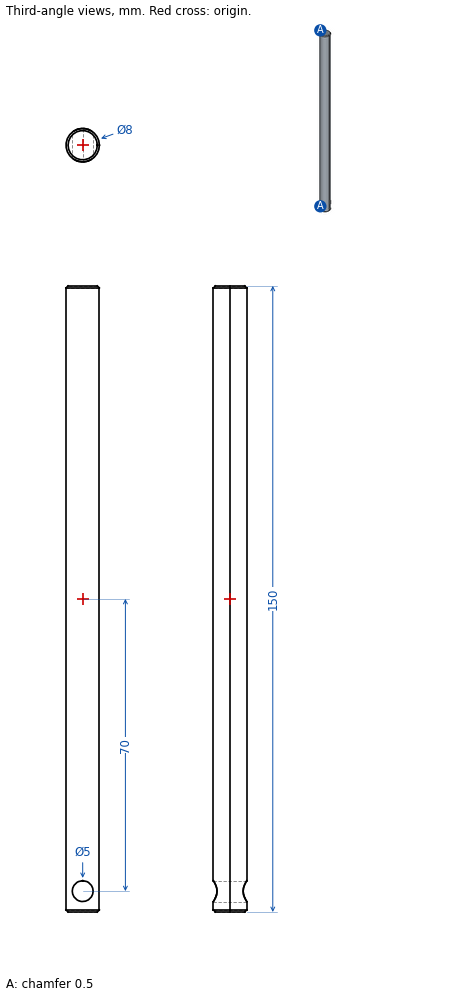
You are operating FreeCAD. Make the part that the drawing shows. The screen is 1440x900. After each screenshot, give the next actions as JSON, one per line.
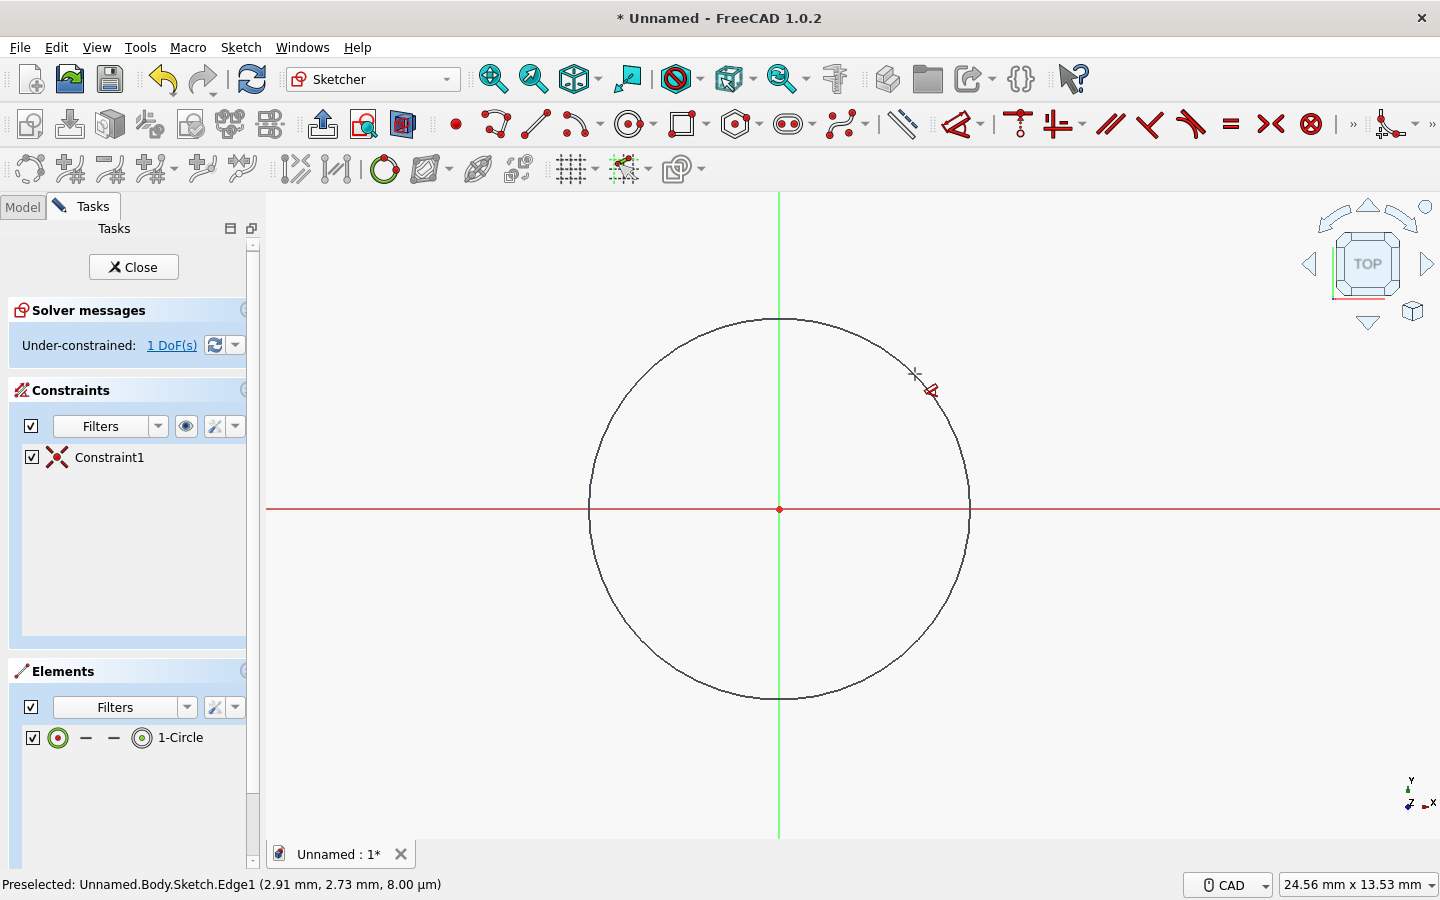
{"action": "left_click", "coordinate": [914, 374]}
{"action": "left_click", "coordinate": [937, 351]}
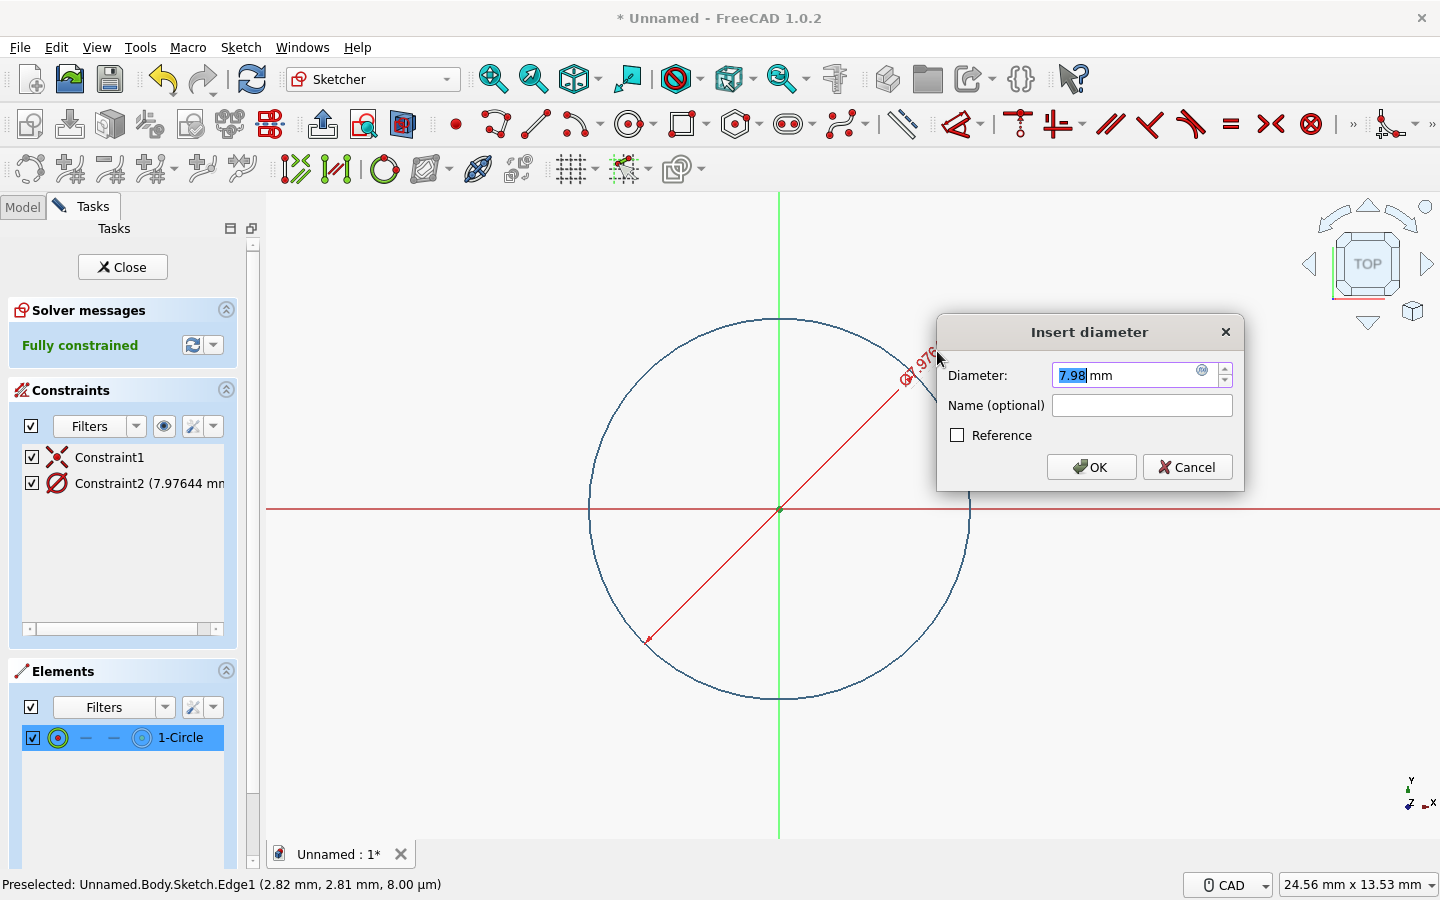
{"action": "type", "text": "8"}
{"action": "key", "text": "Return"}
{"action": "key", "text": "Escape"}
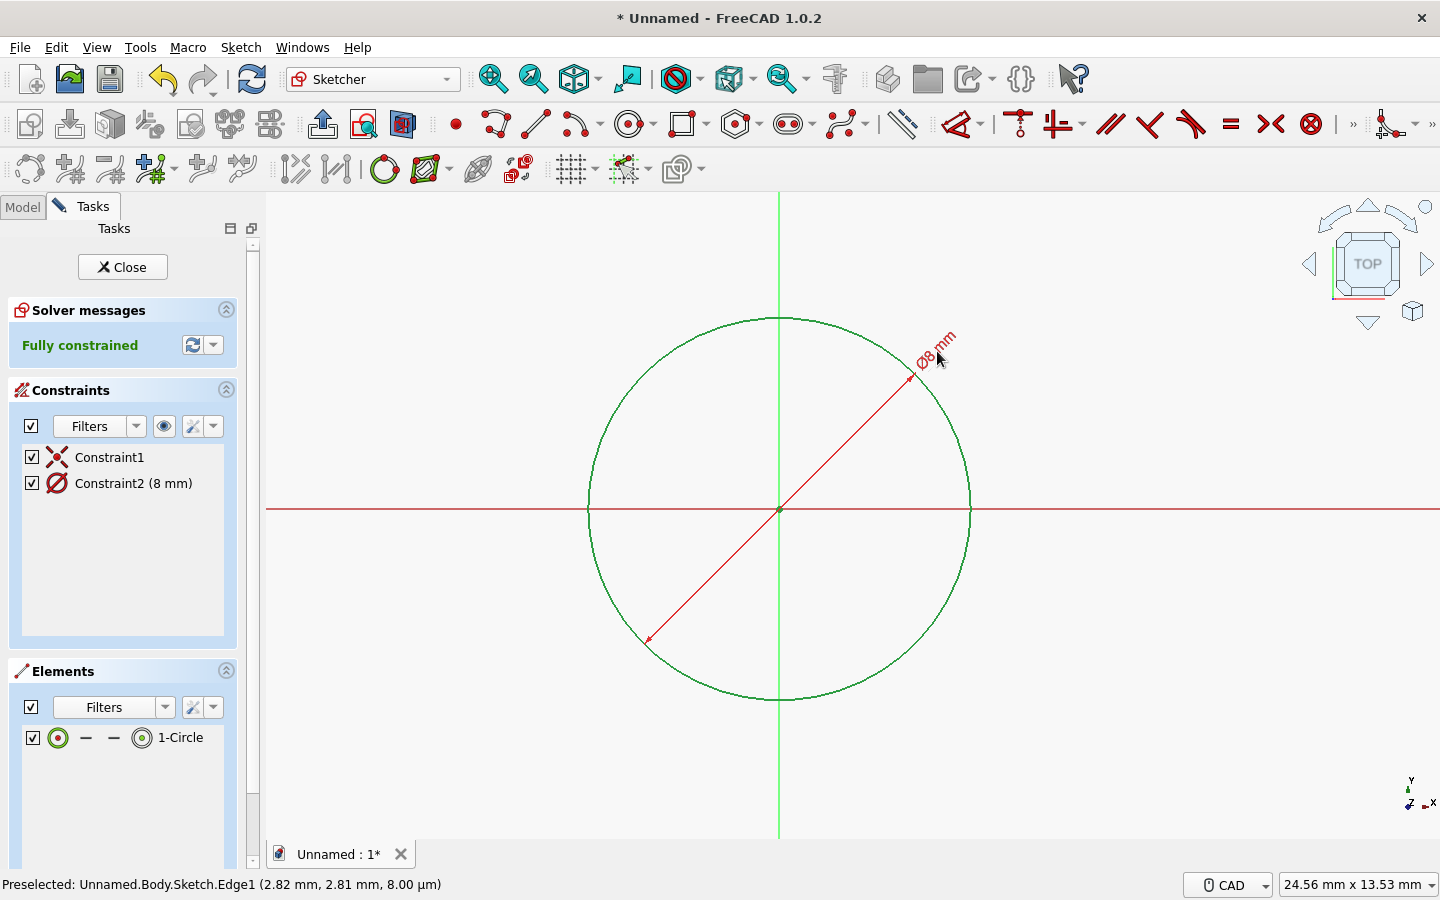
{"action": "left_click", "coordinate": [123, 267]}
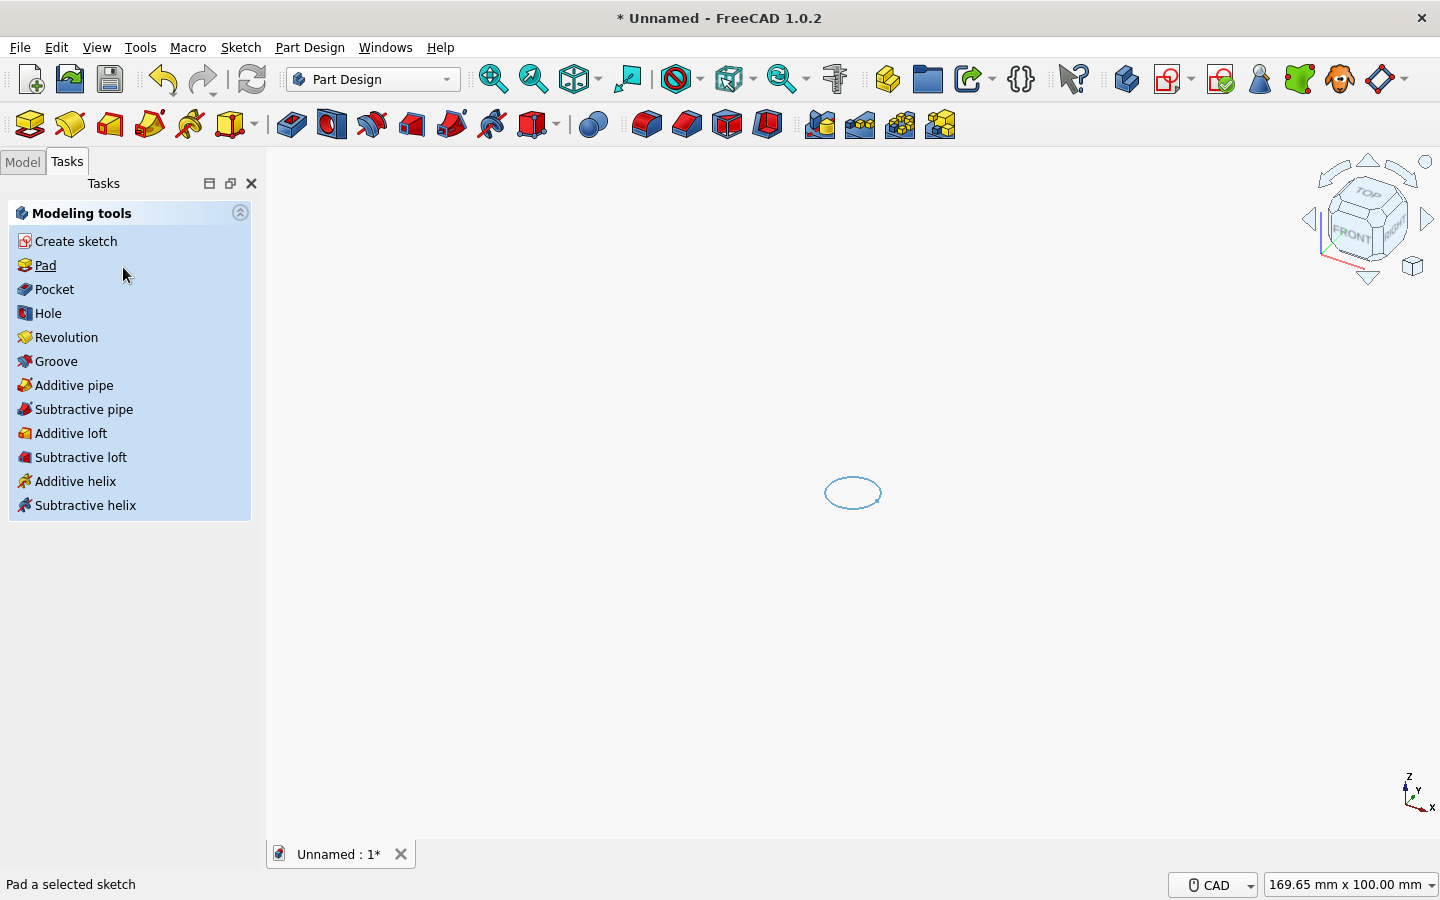
{"action": "left_click", "coordinate": [30, 124]}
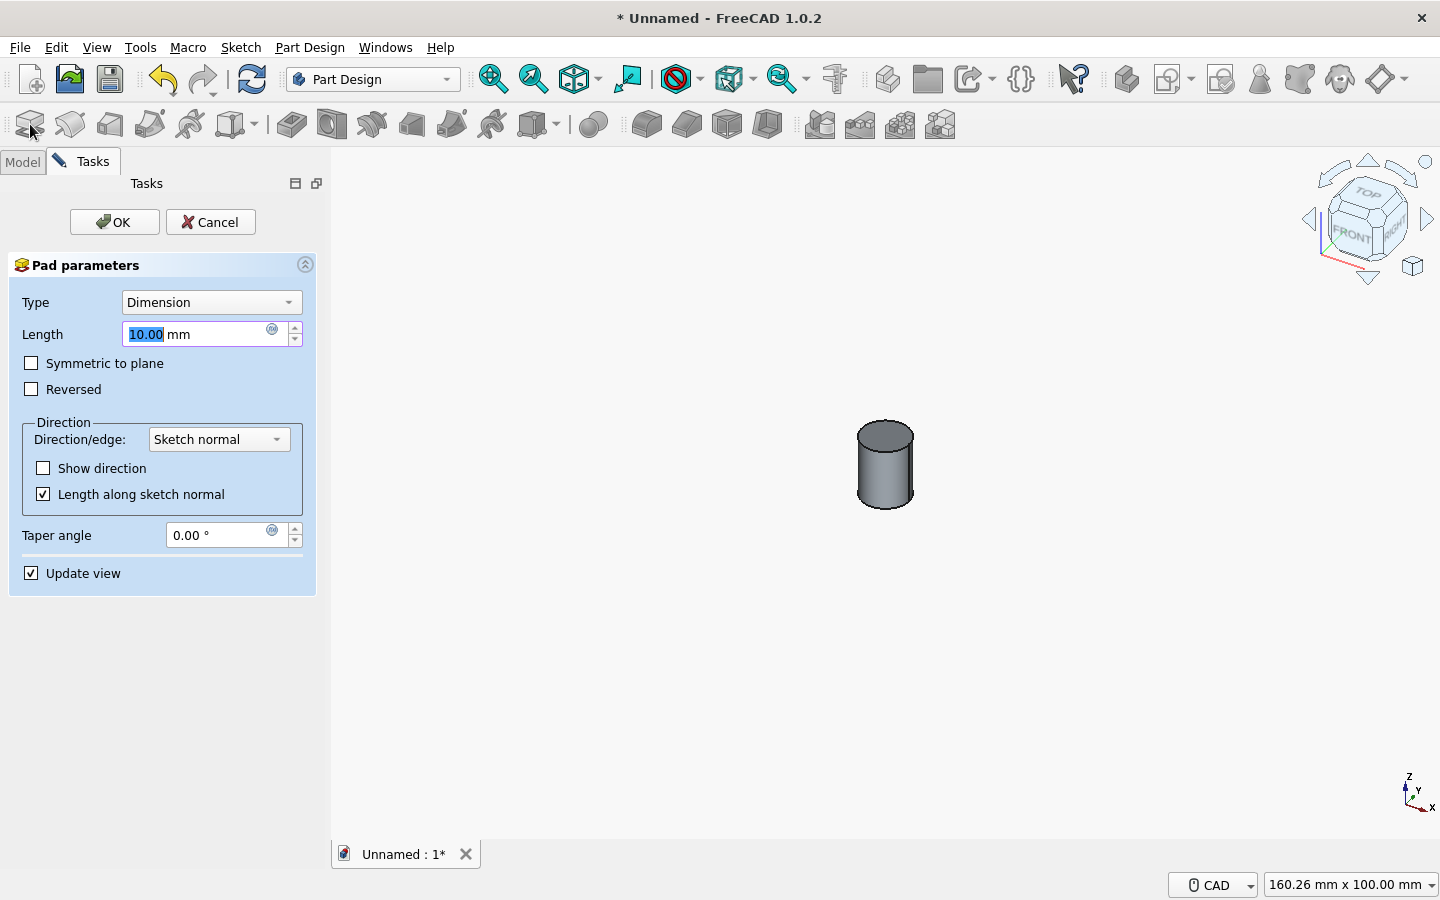
{"action": "type", "text": "150"}
{"action": "key", "text": "Tab"}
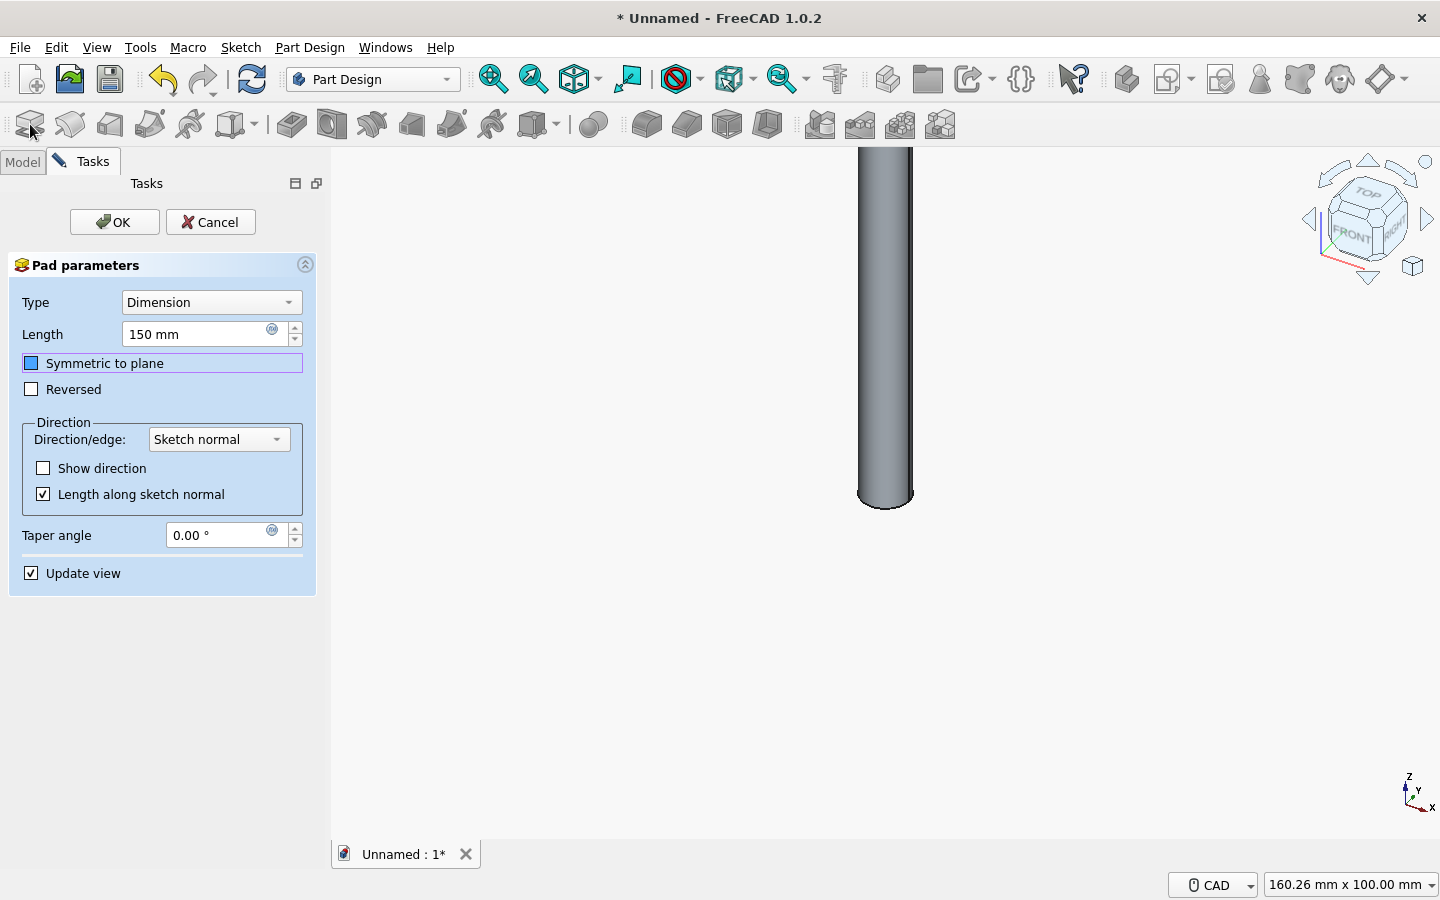
{"action": "left_click", "coordinate": [30, 363]}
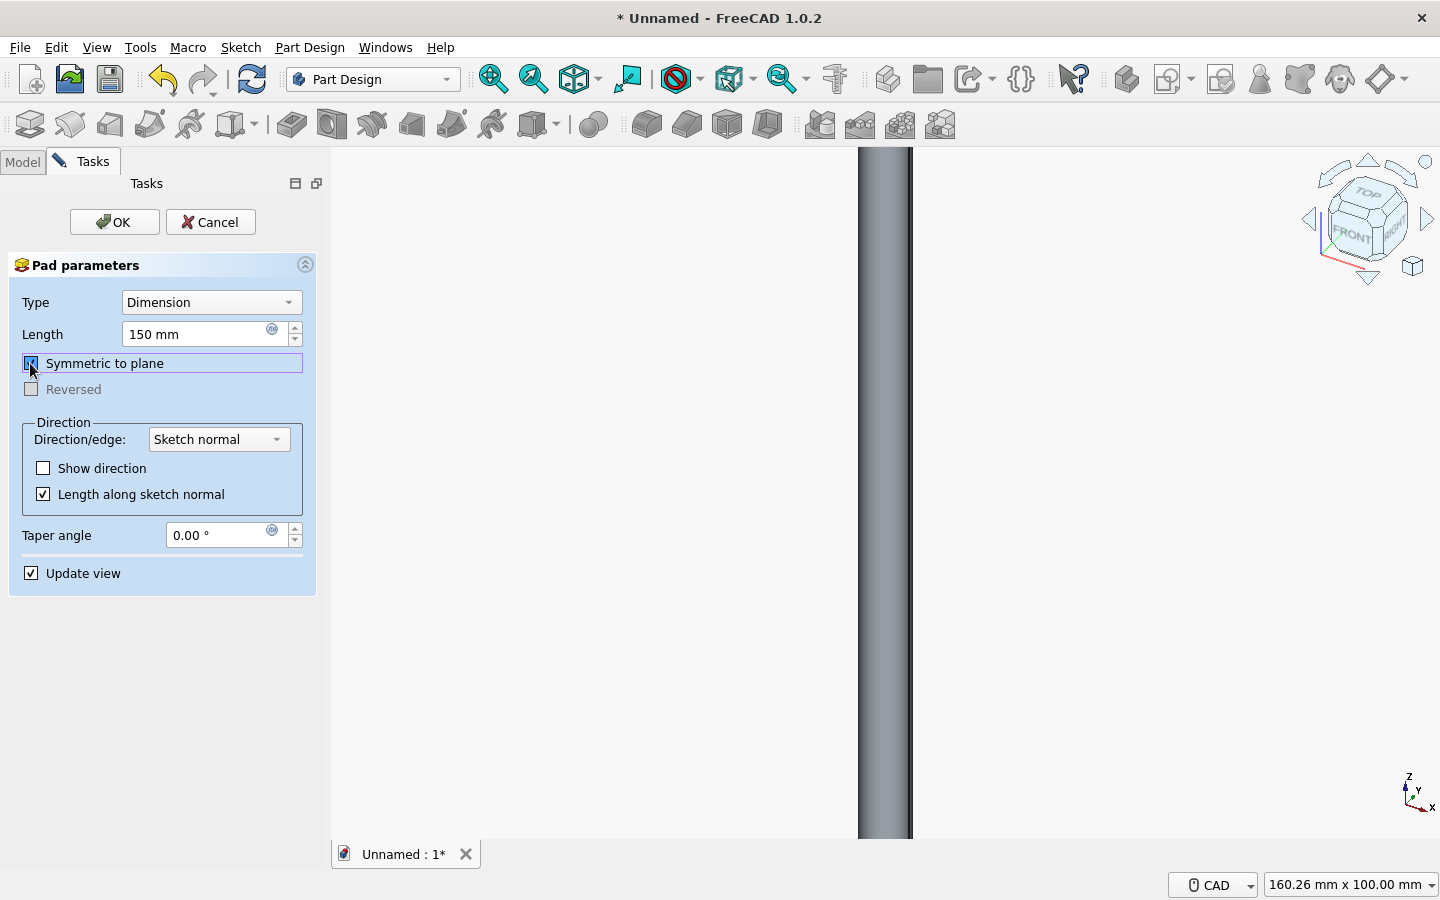
{"action": "left_click", "coordinate": [115, 222]}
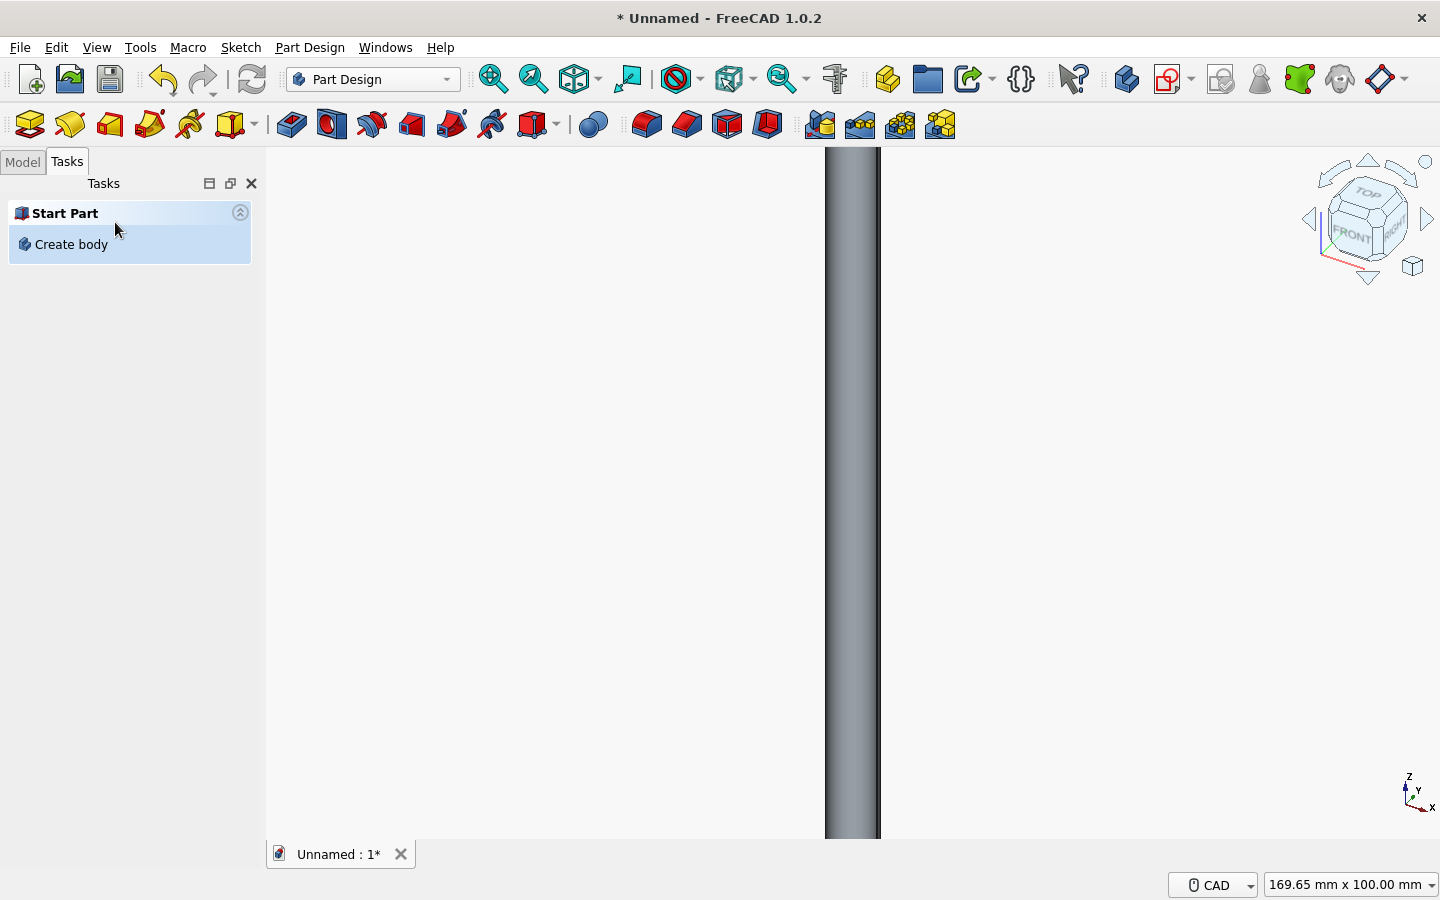
{"action": "key", "text": "v f"}